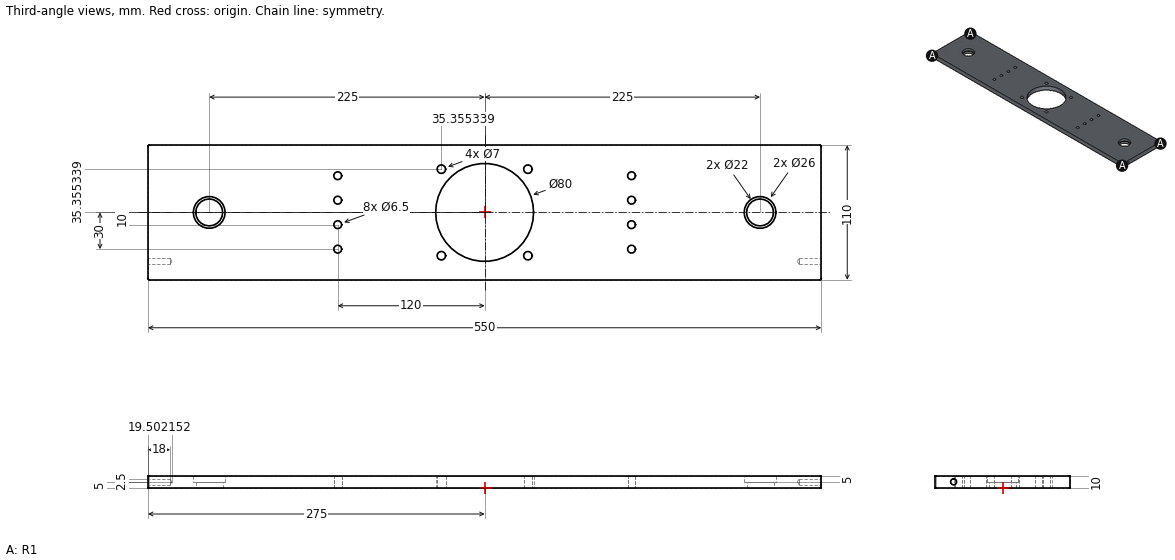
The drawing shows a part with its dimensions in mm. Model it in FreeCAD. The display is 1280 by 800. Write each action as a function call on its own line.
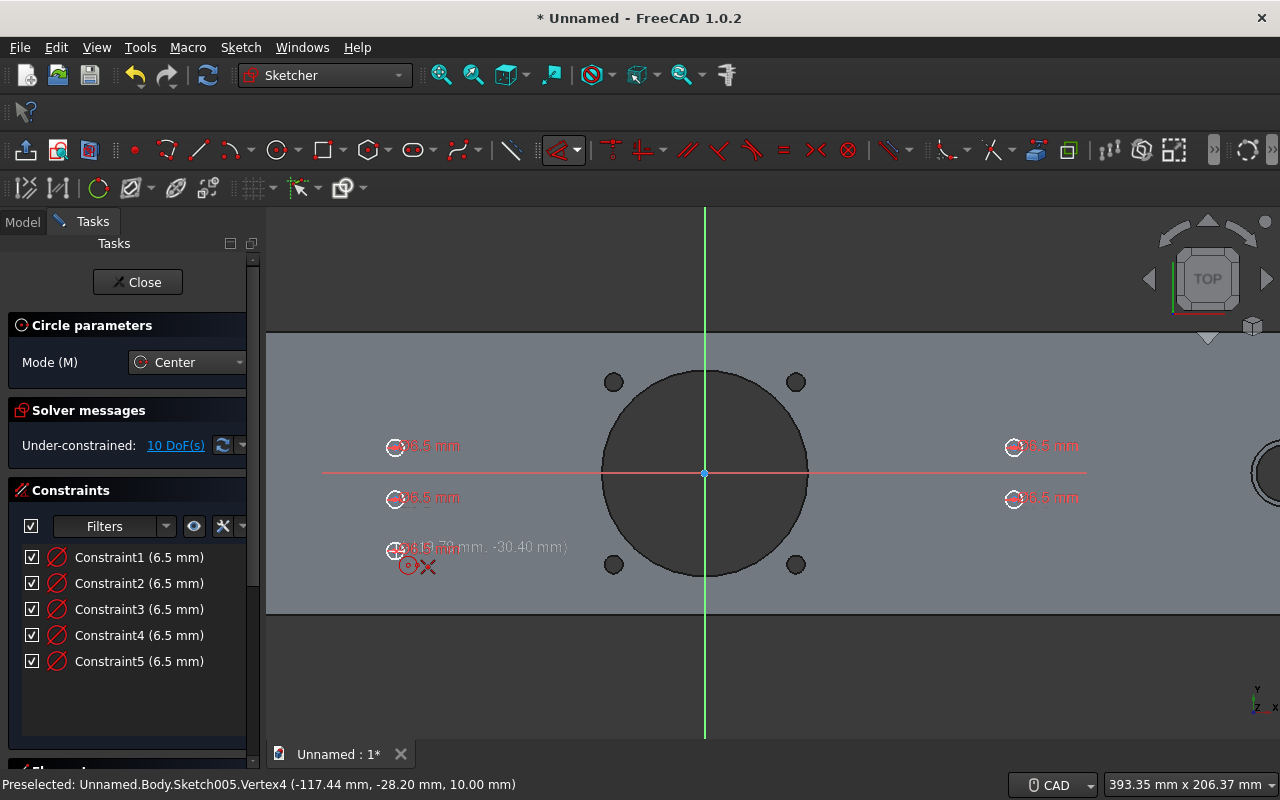
scroll(396, 396, up, 5)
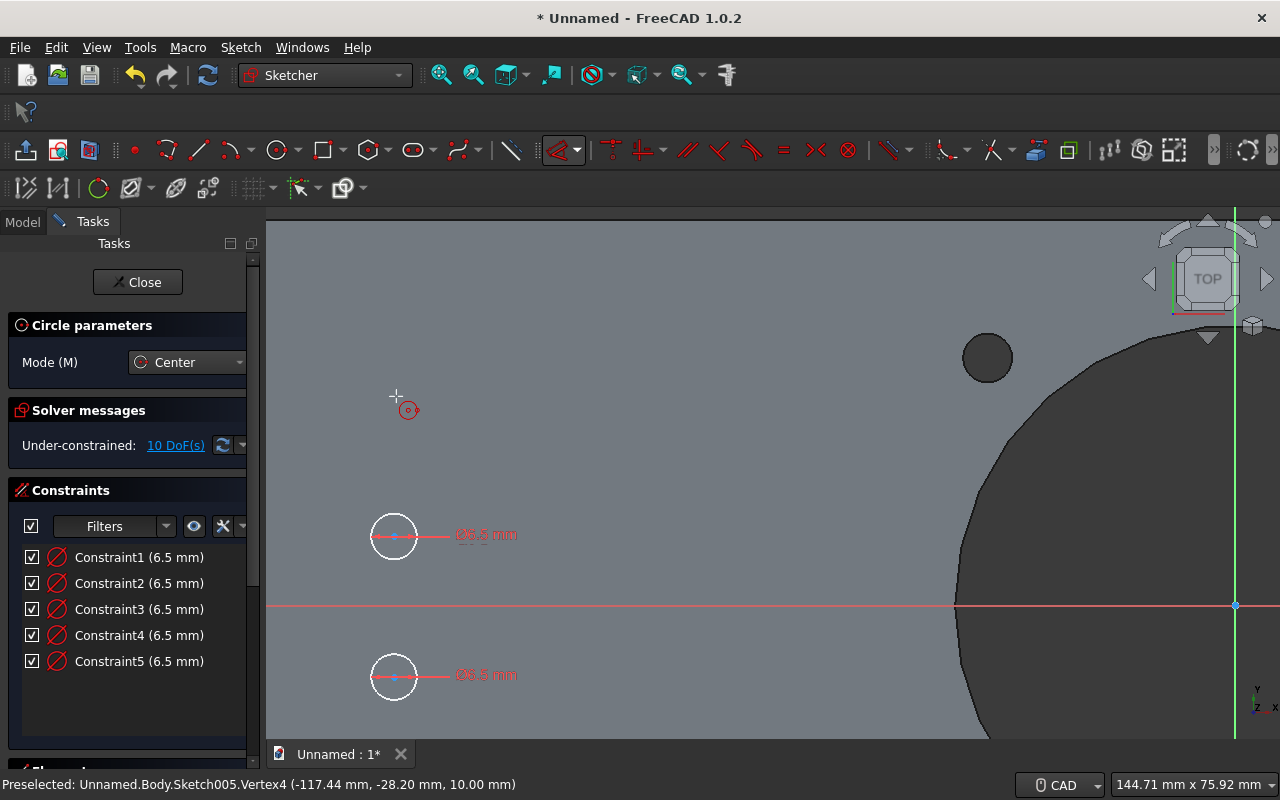
click(394, 396)
move(411, 379)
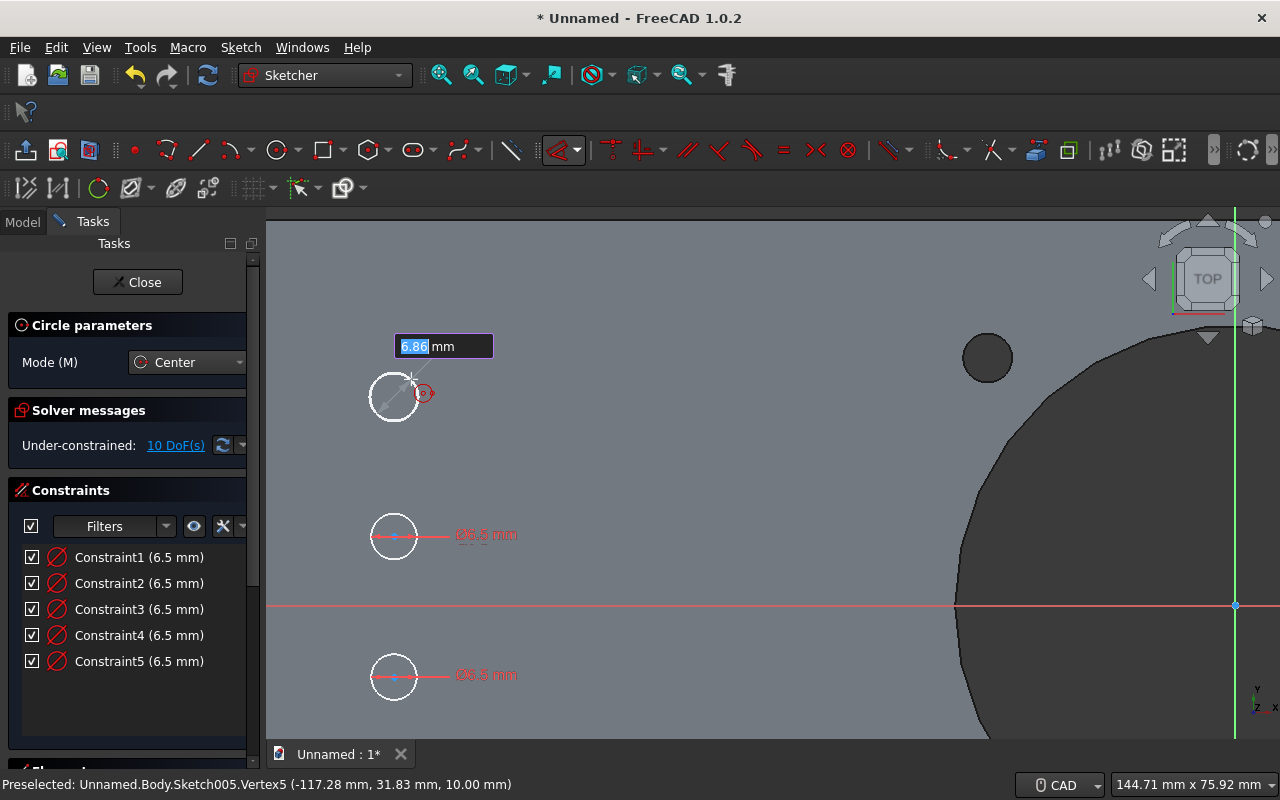
text(6.5)
key(Return)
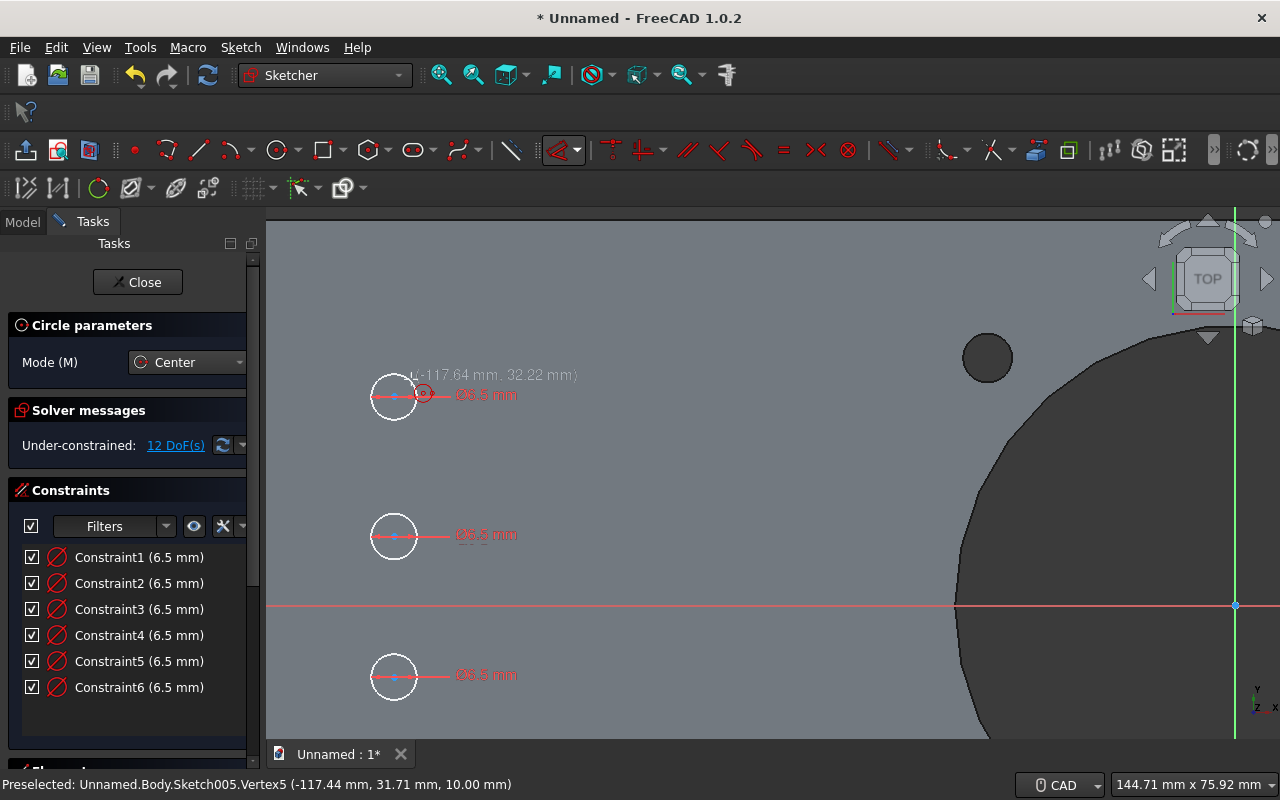
scroll(396, 396, down, 5)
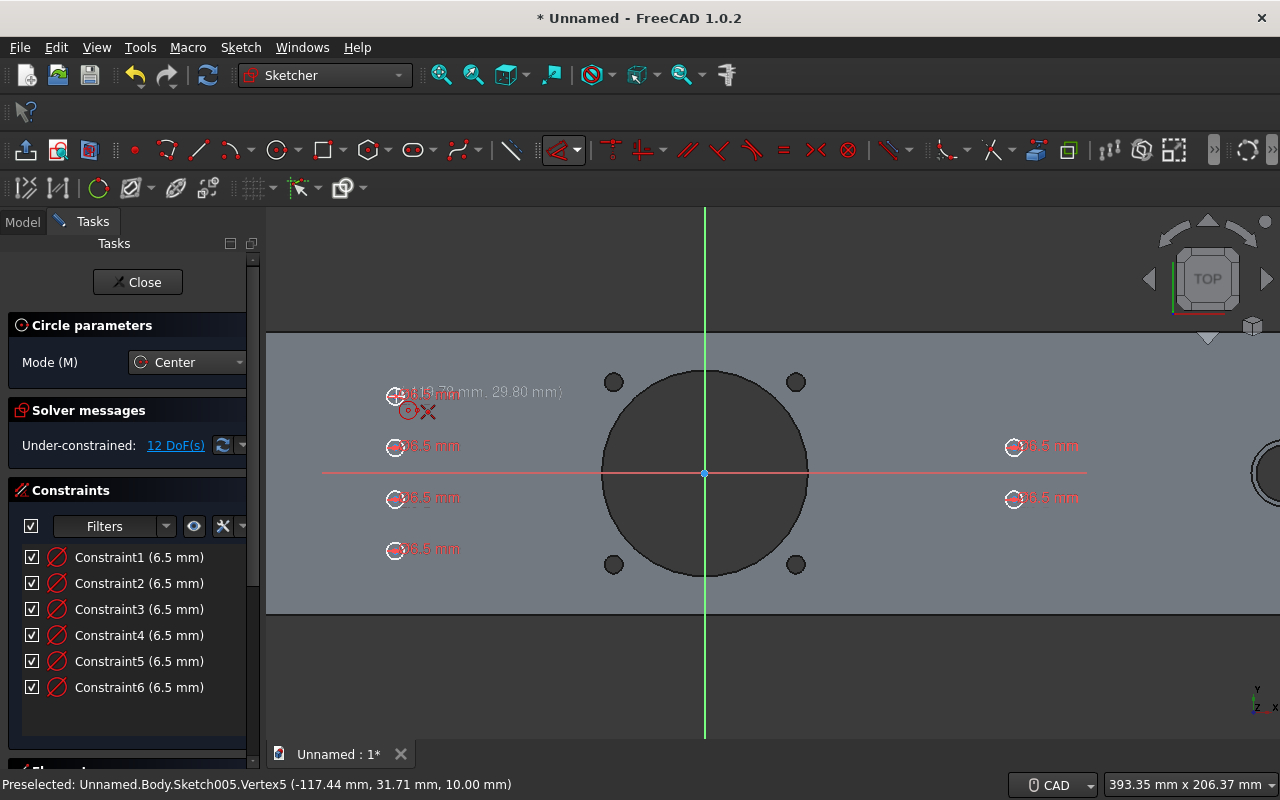
scroll(1014, 396, up, 5)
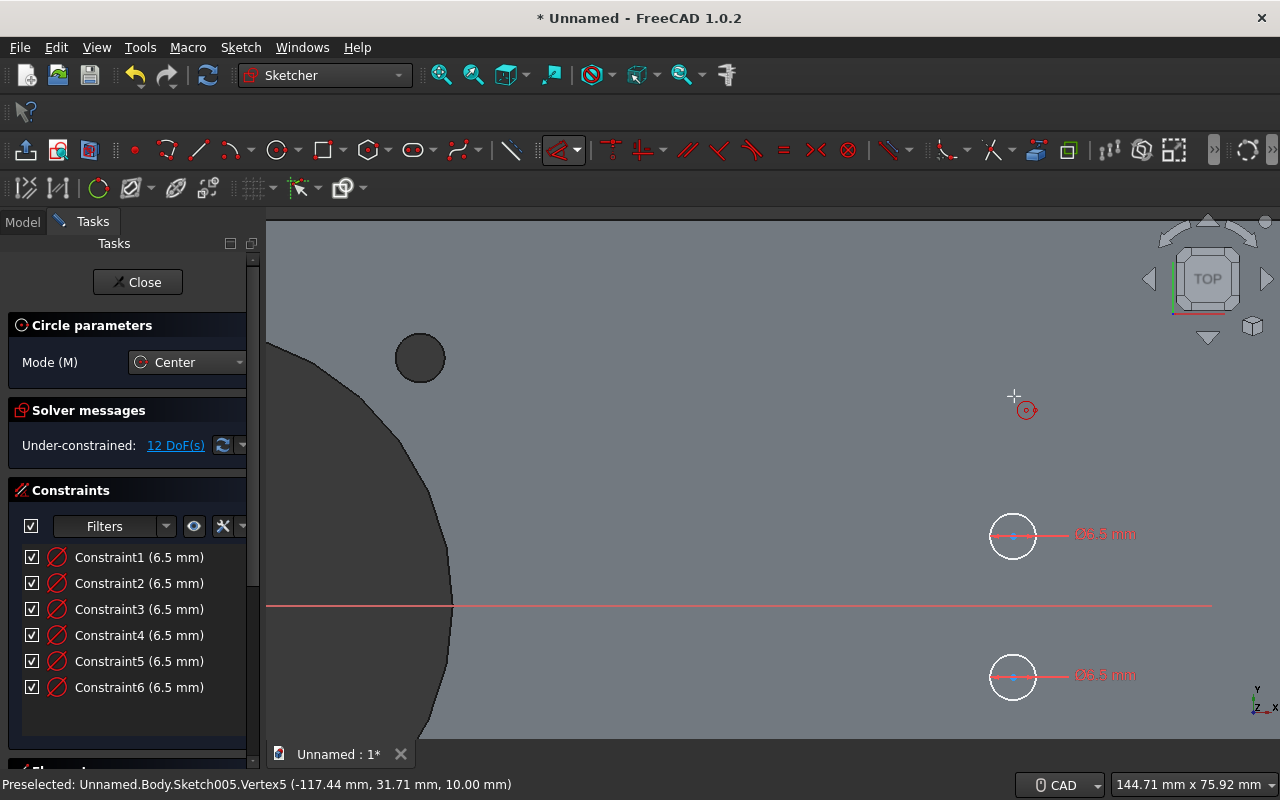
click(1013, 396)
move(1029, 379)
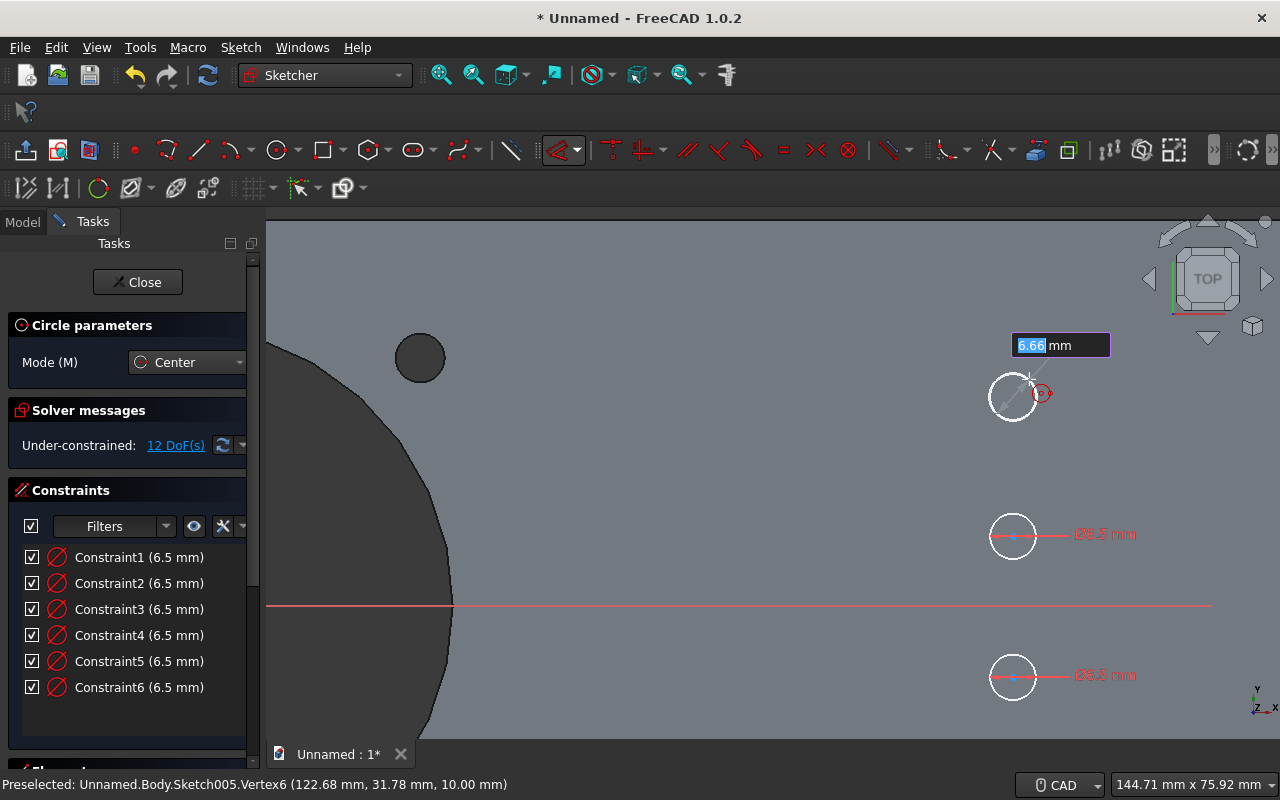
text(6.5)
key(Return)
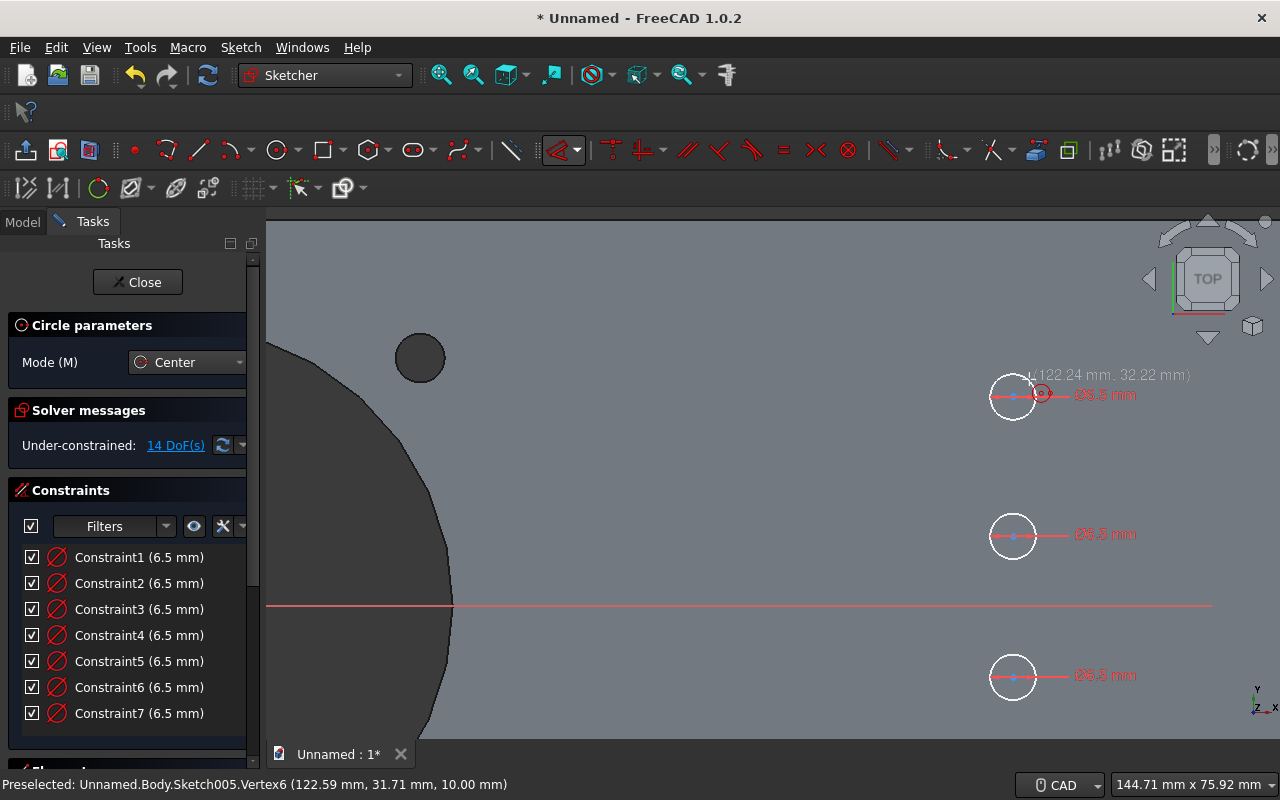
scroll(1014, 396, down, 5)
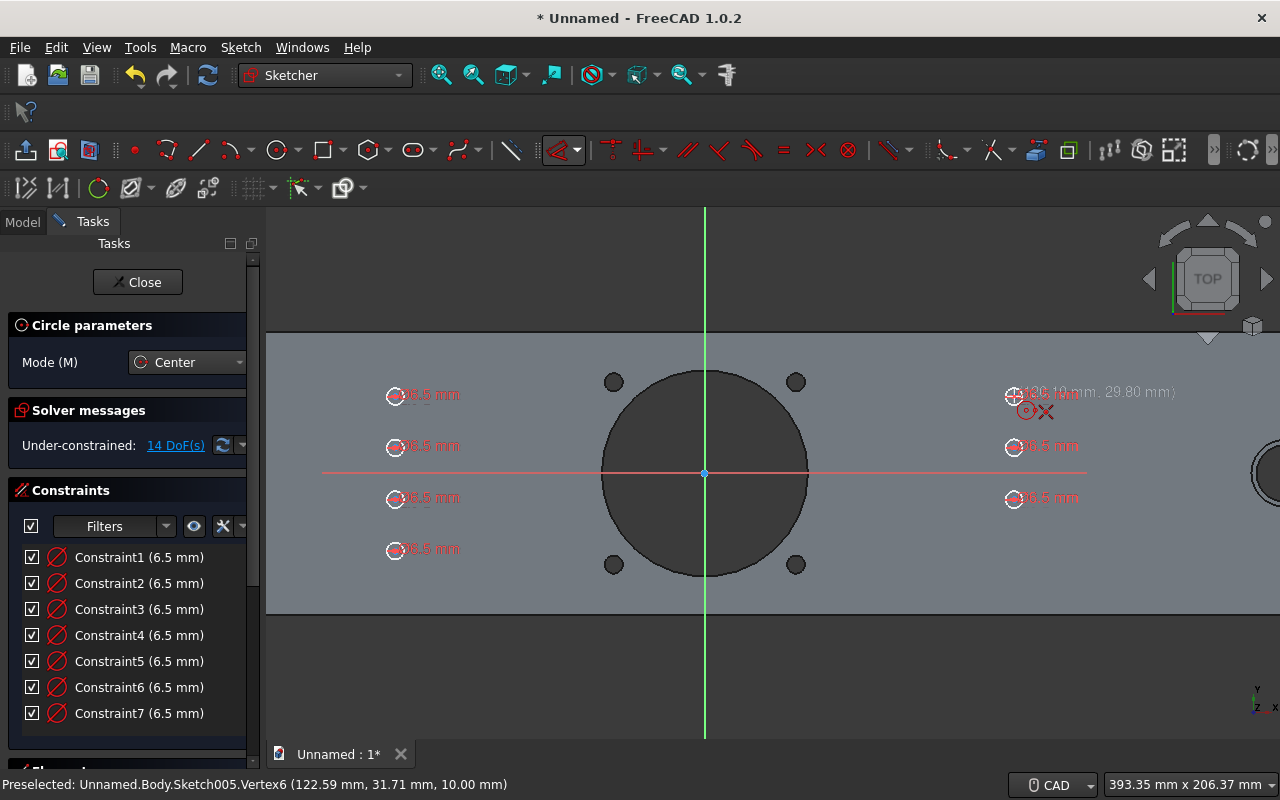
scroll(1014, 551, up, 5)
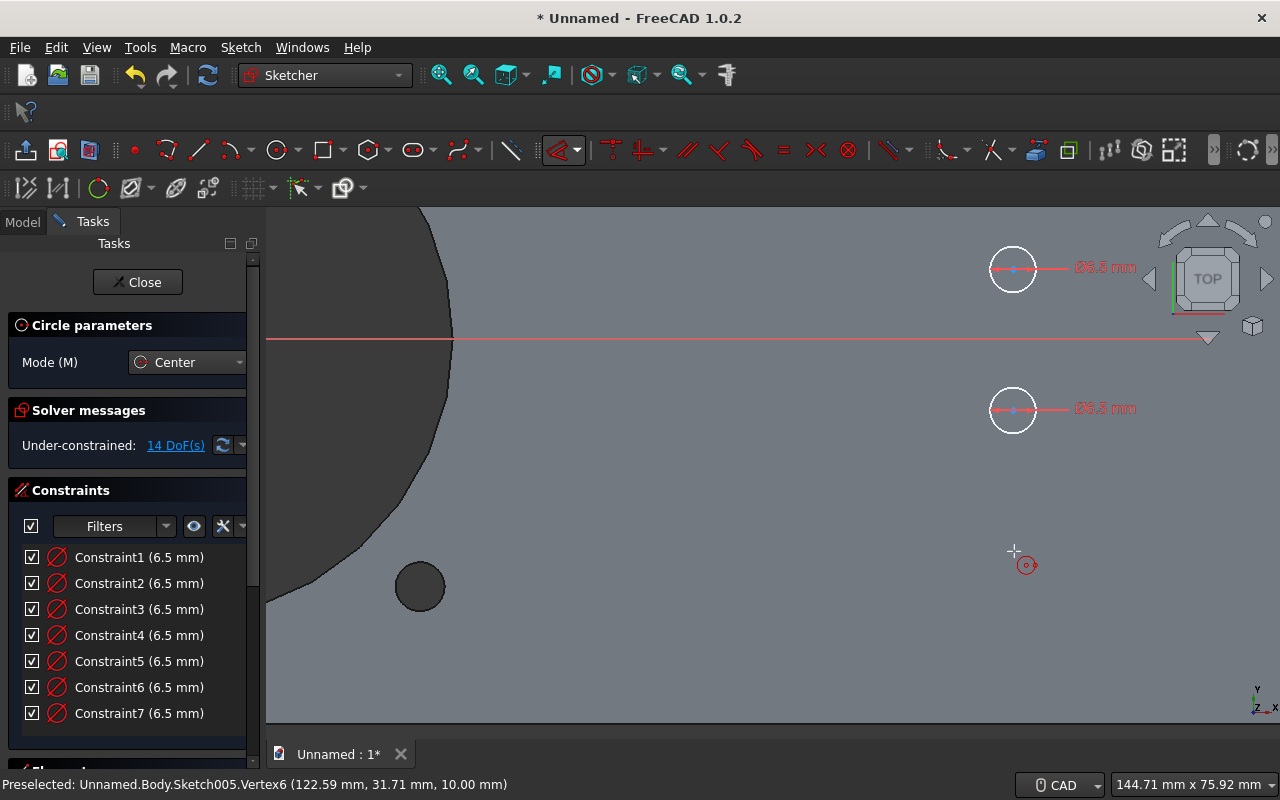
click(1013, 549)
move(1029, 533)